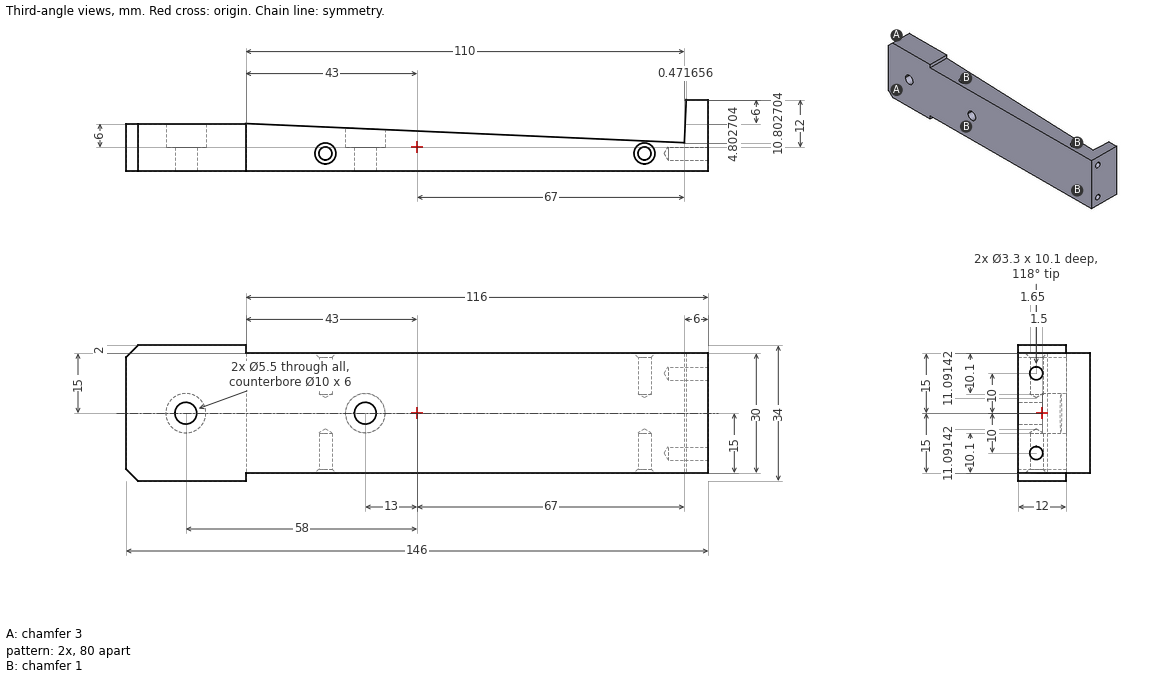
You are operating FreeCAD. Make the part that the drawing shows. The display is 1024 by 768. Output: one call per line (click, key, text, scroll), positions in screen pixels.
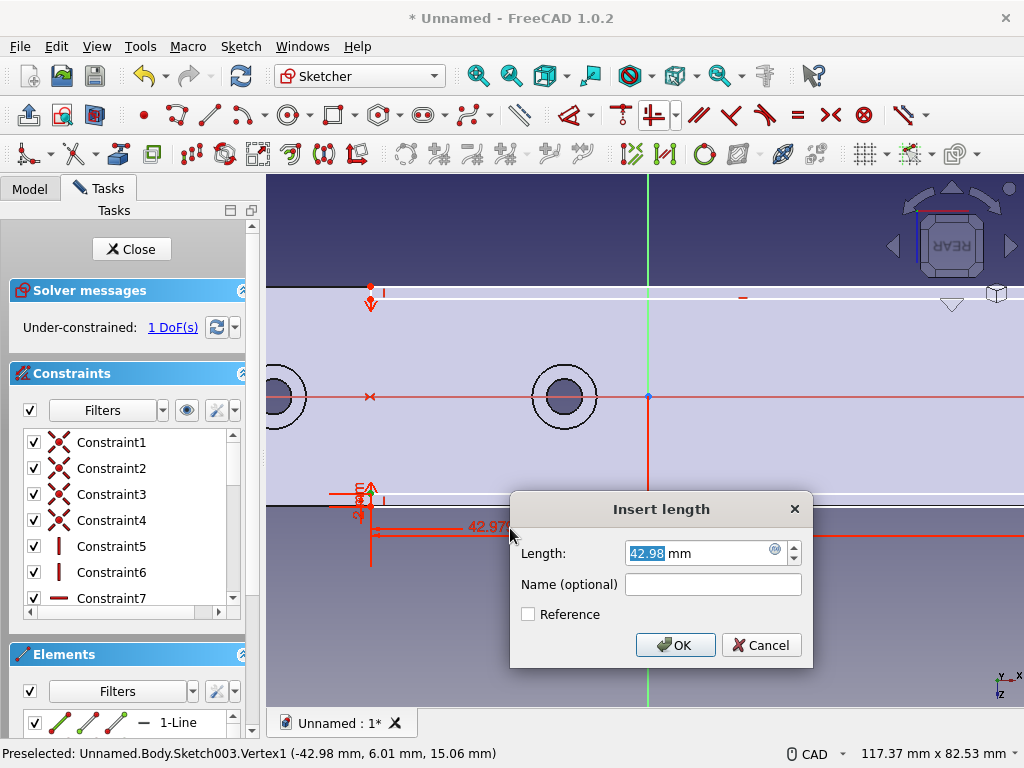
text(43)
key(Return)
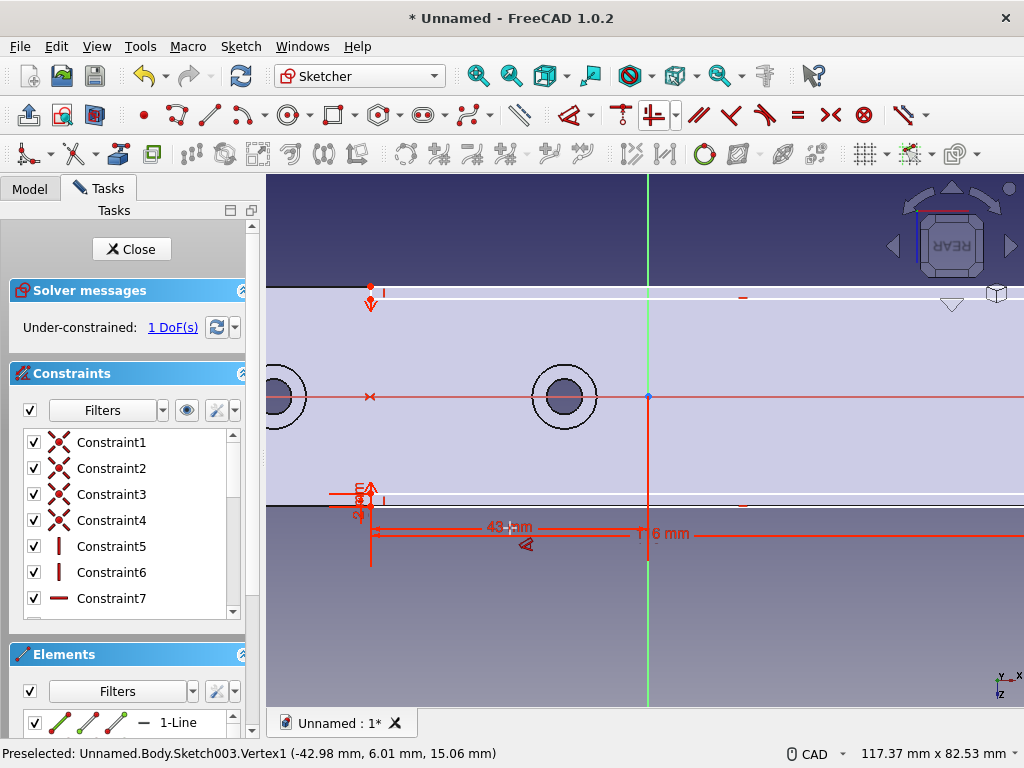
click(371, 494)
click(337, 445)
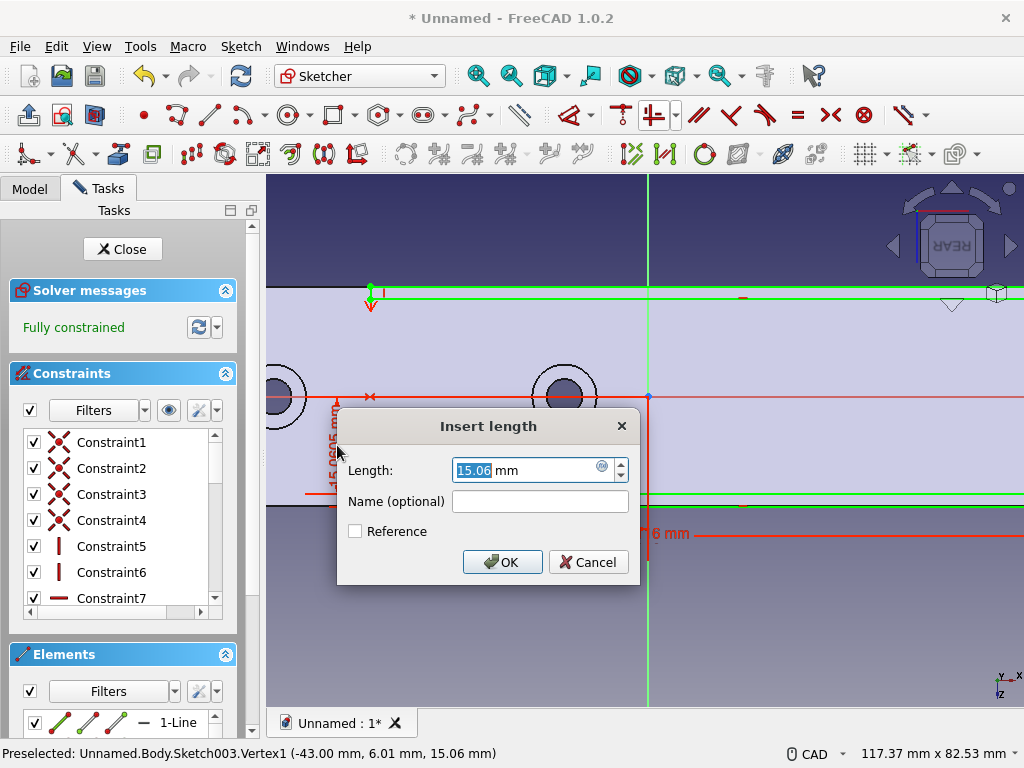
text(15)
key(Return)
key(Escape)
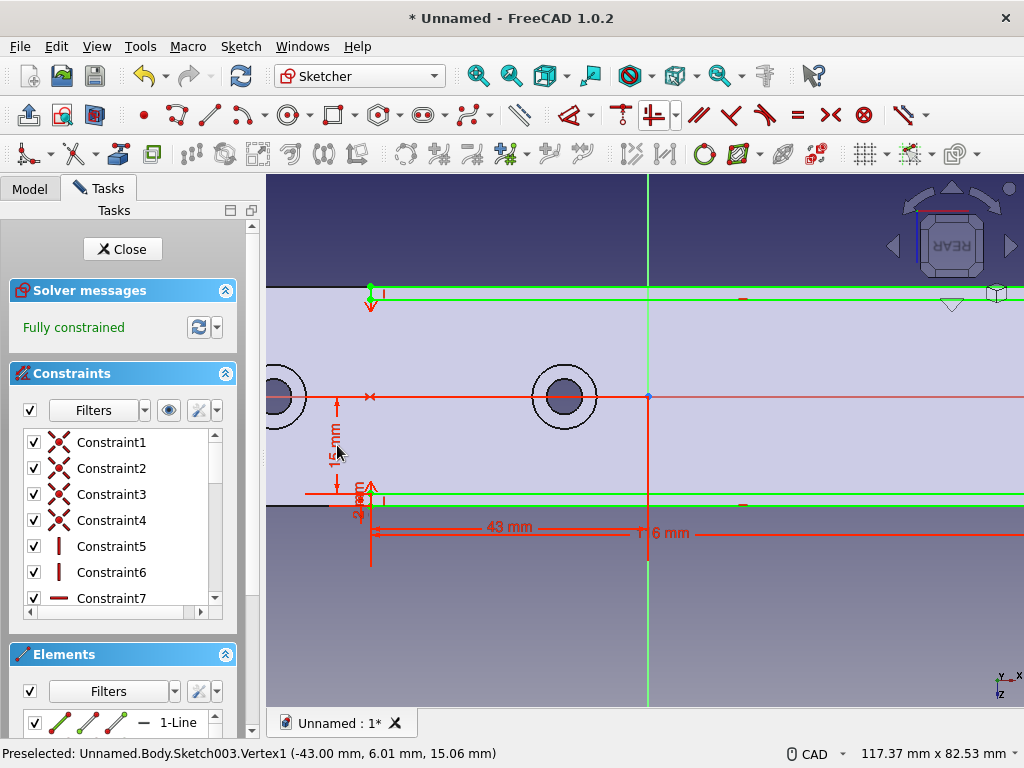
click(123, 249)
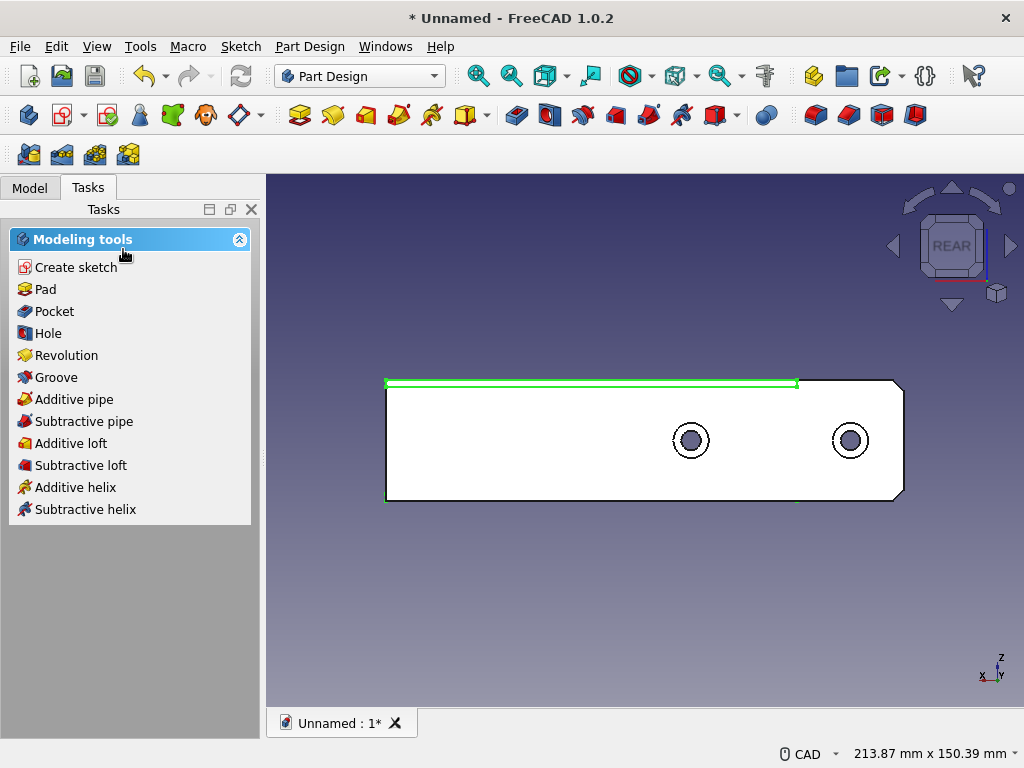
click(517, 116)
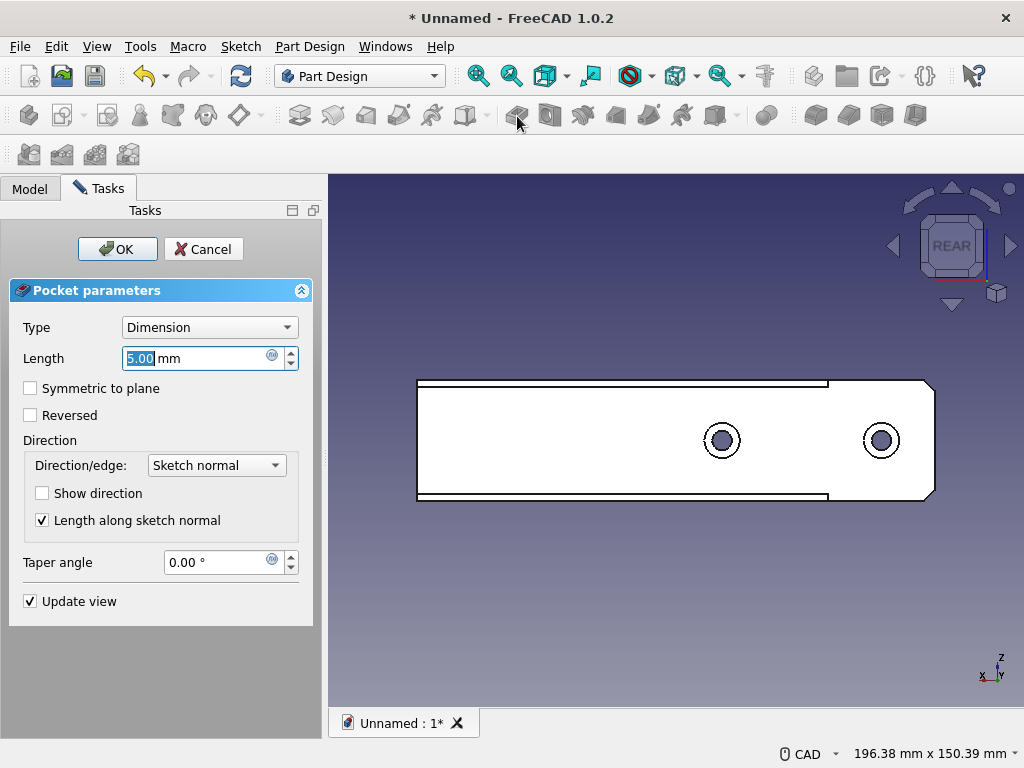
click(210, 328)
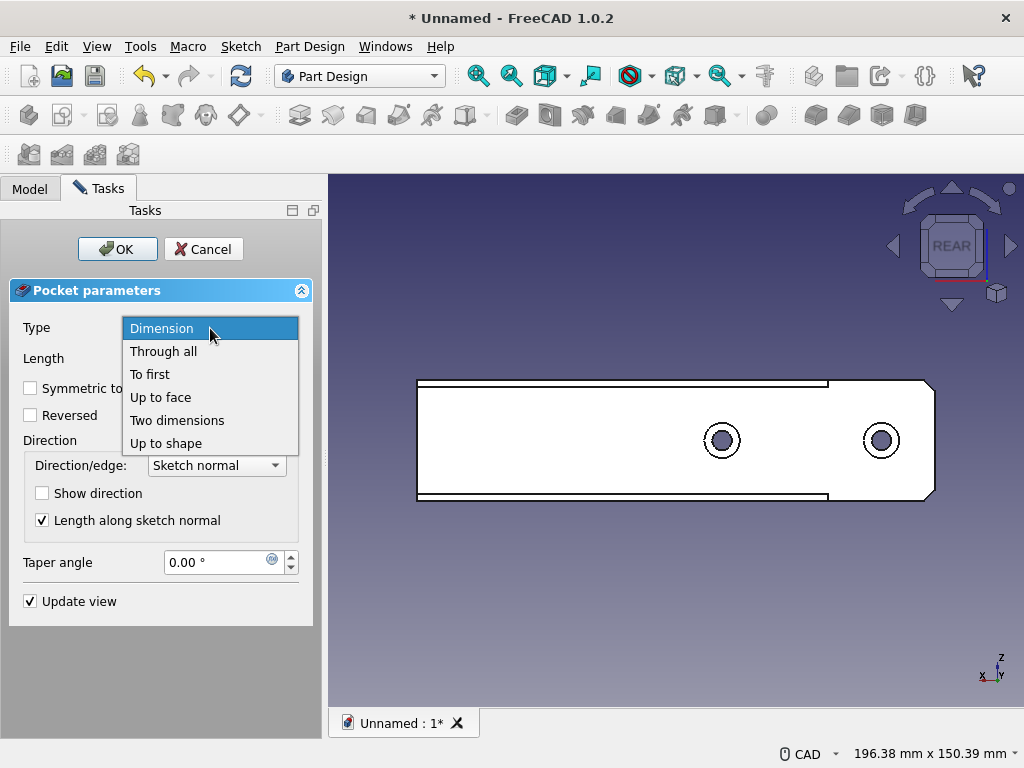
click(208, 352)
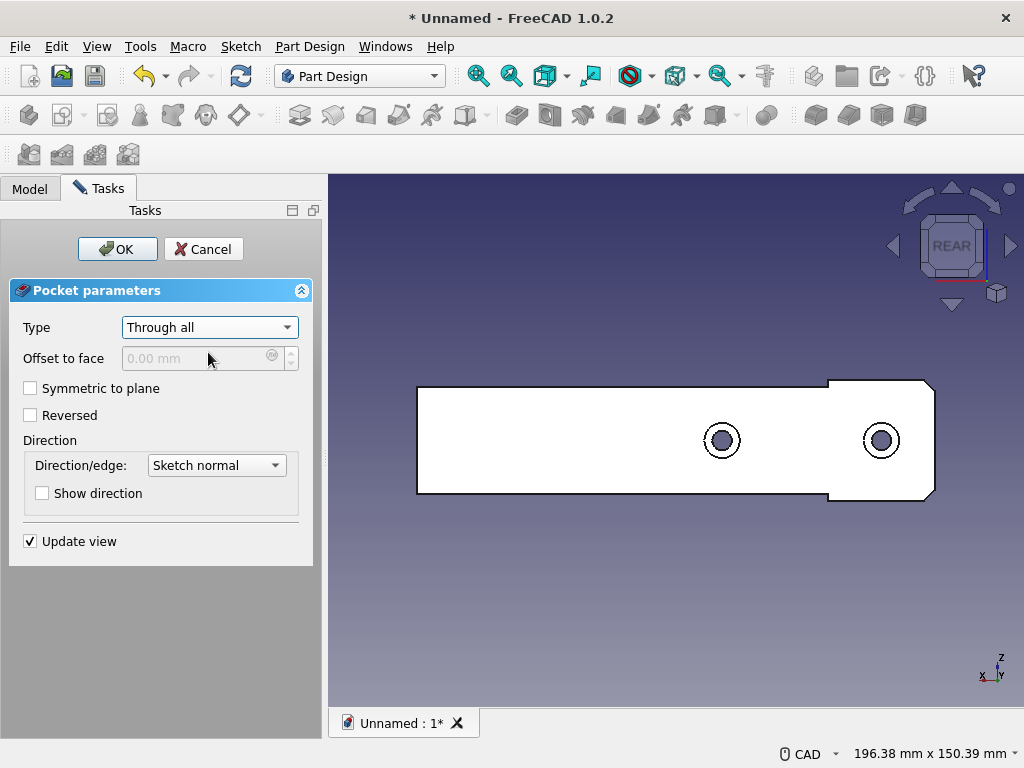
click(118, 249)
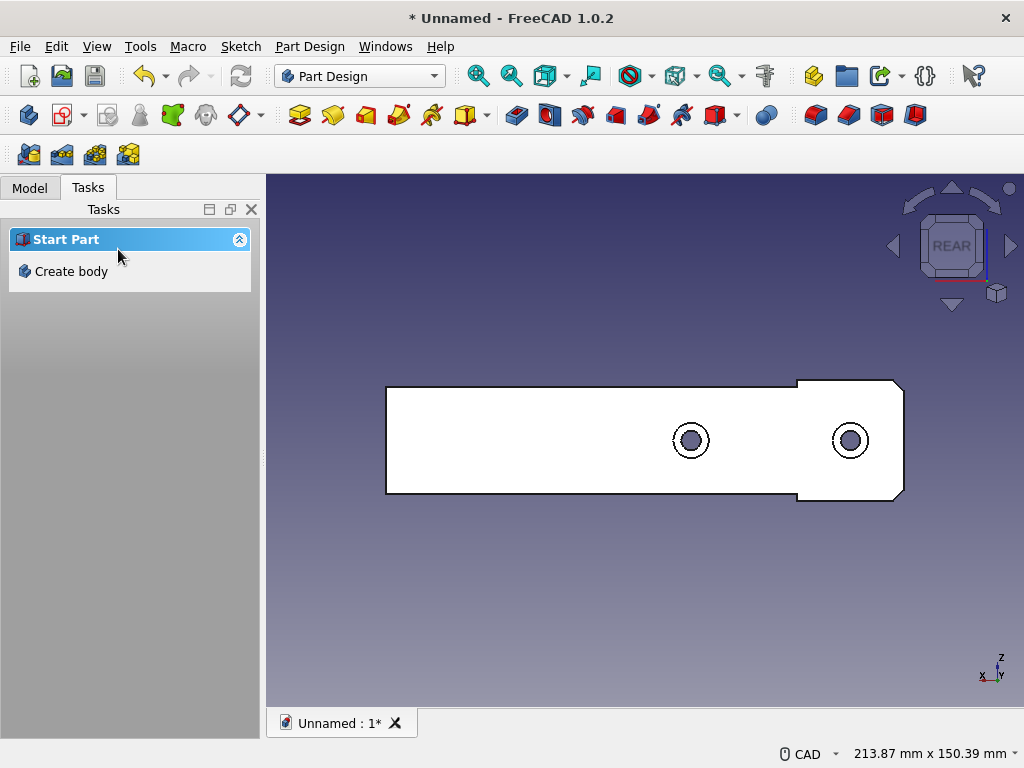
click(30, 188)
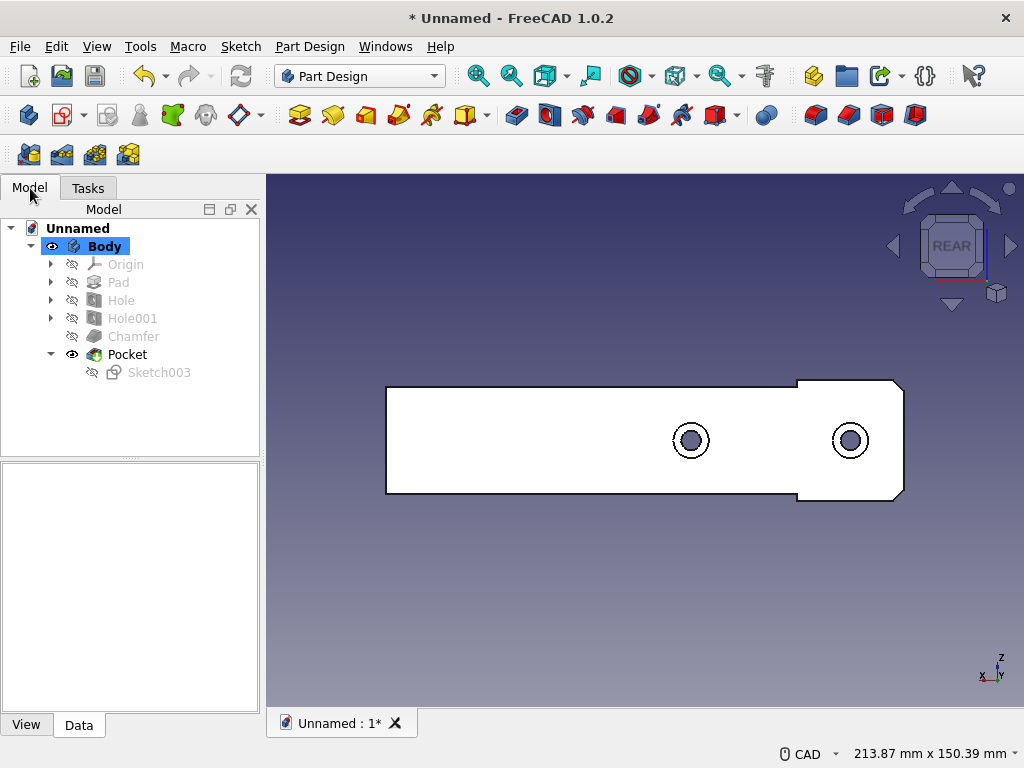
click(51, 264)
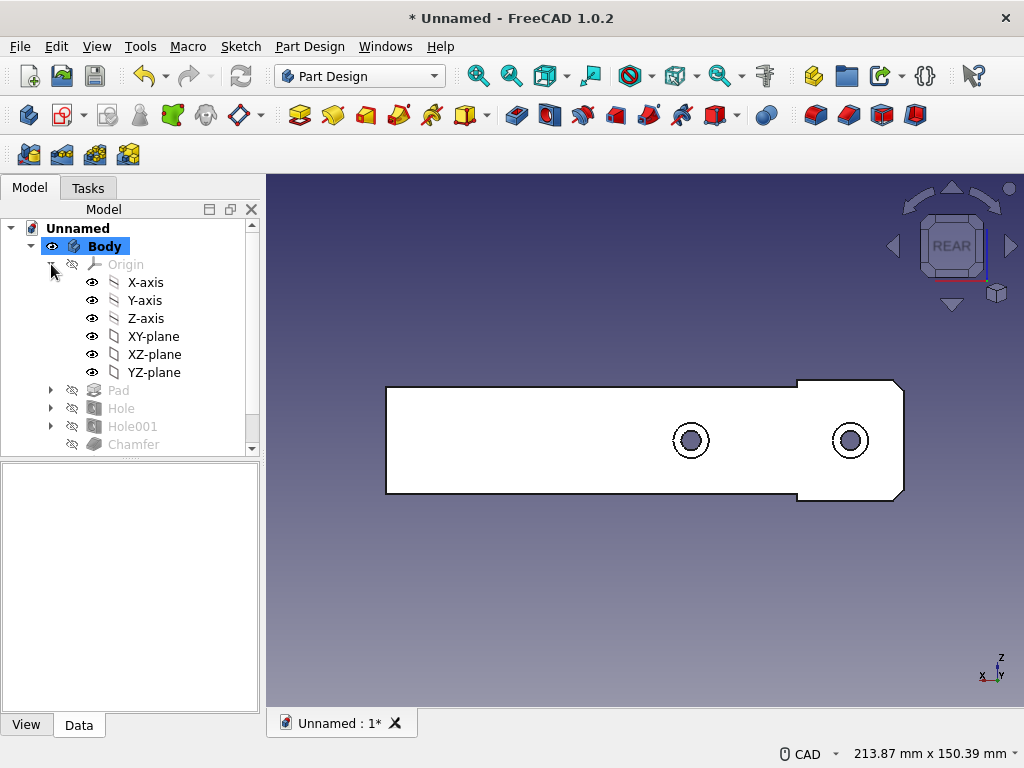
click(137, 372)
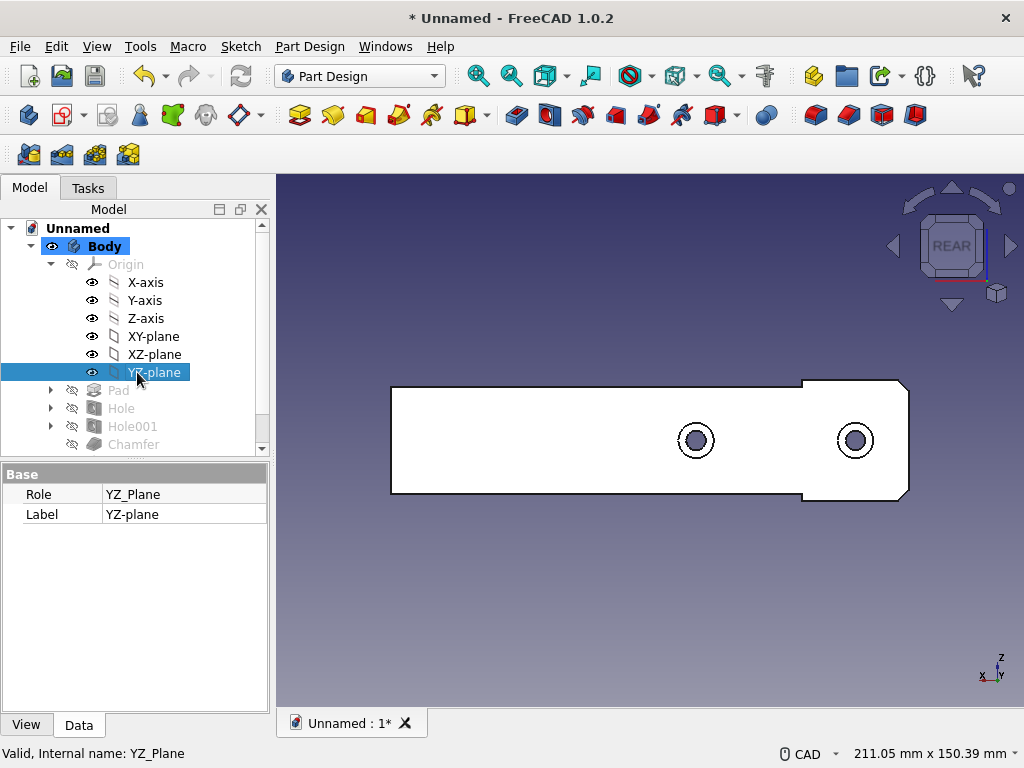
click(238, 116)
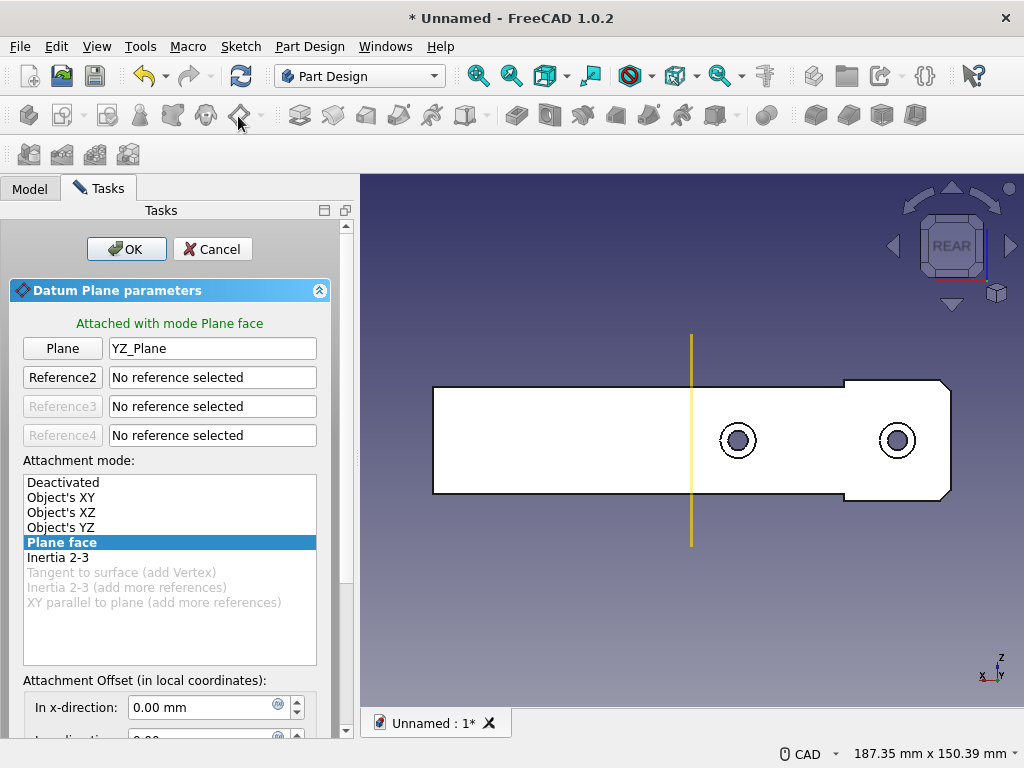
scroll(346, 479, down, 2)